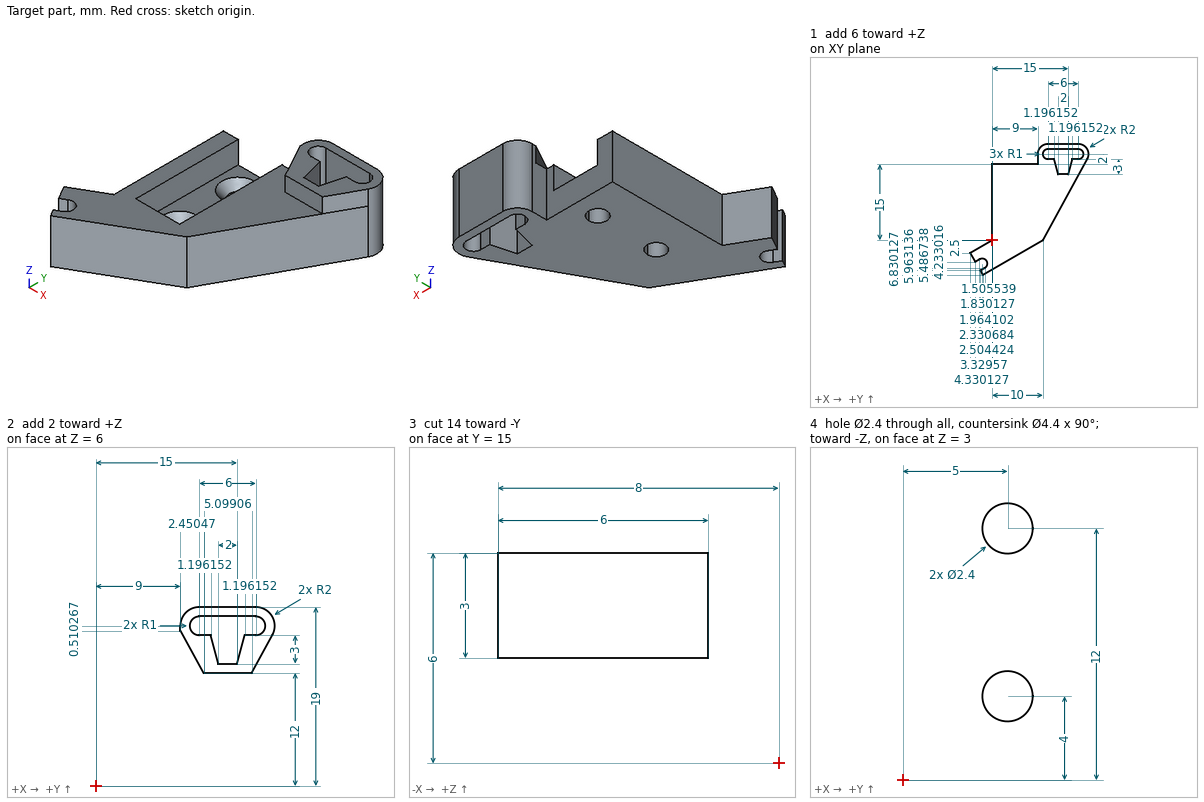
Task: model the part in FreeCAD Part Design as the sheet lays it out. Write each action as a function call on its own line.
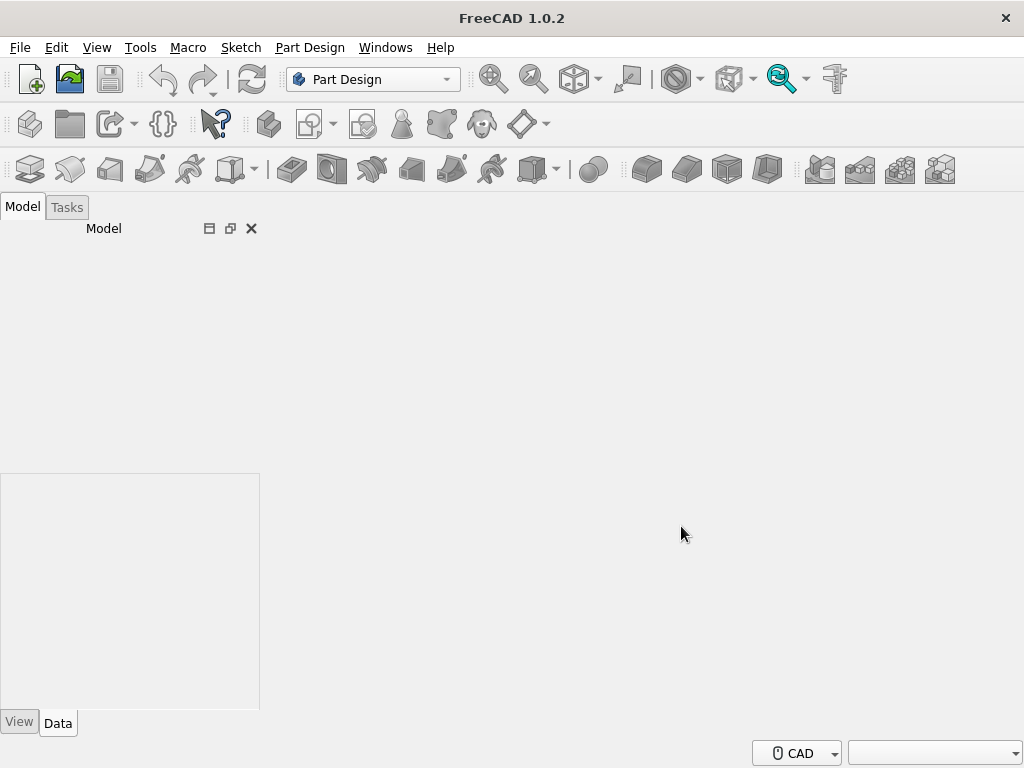
click(30, 80)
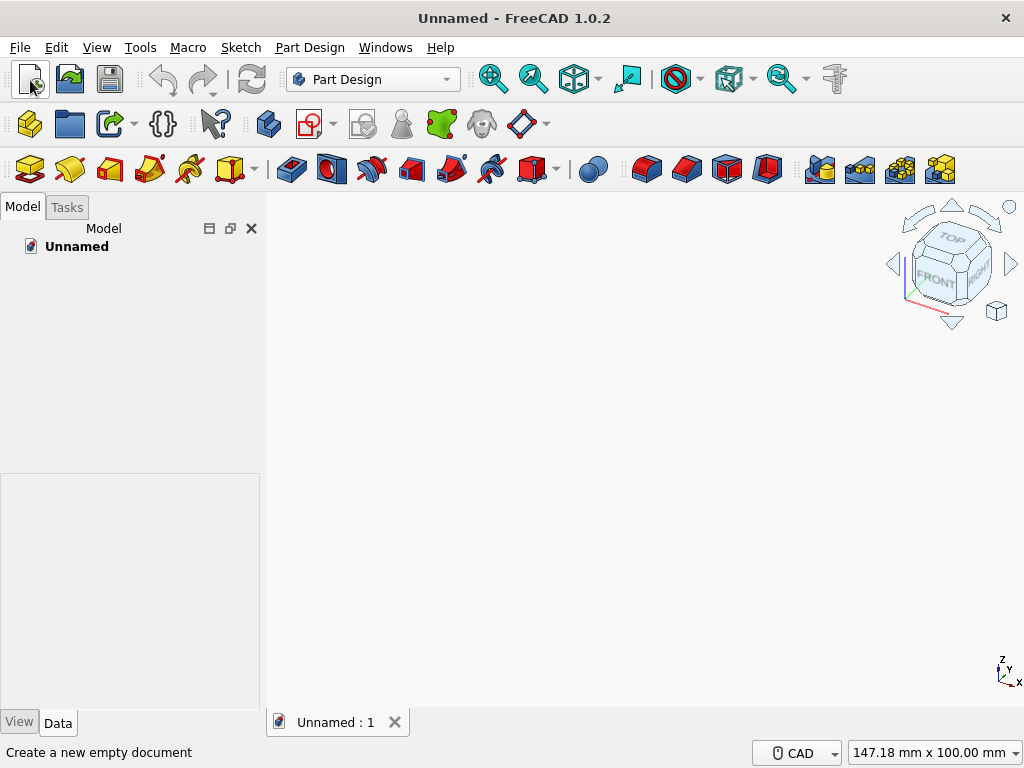
click(310, 124)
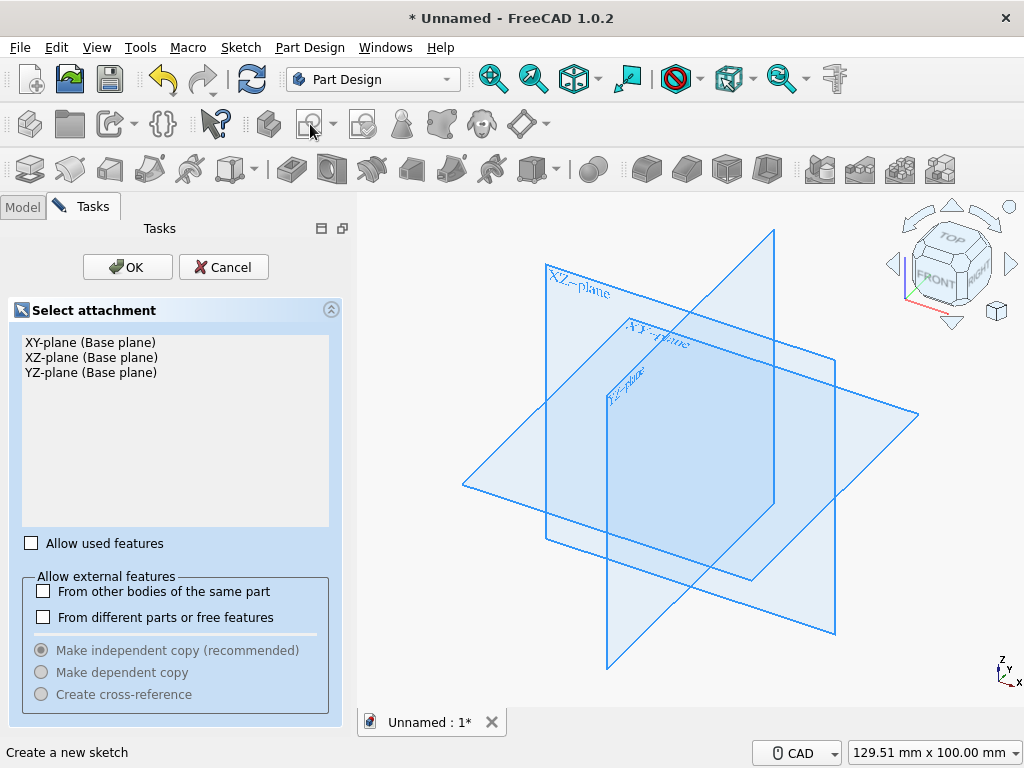
click(82, 342)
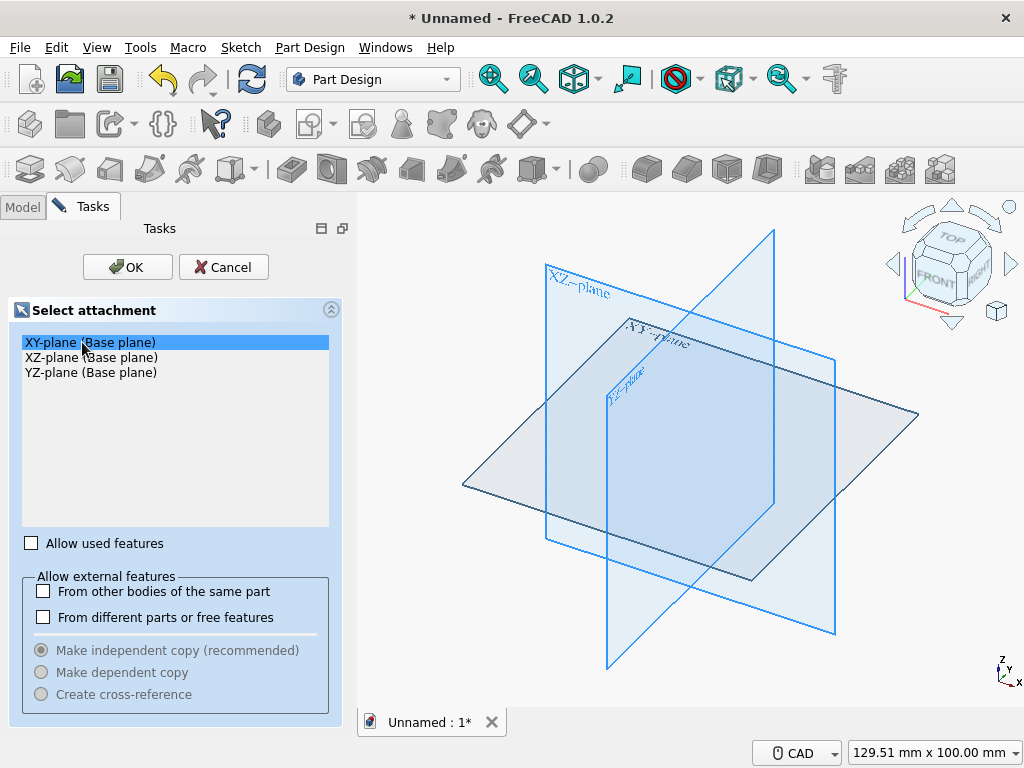
click(128, 267)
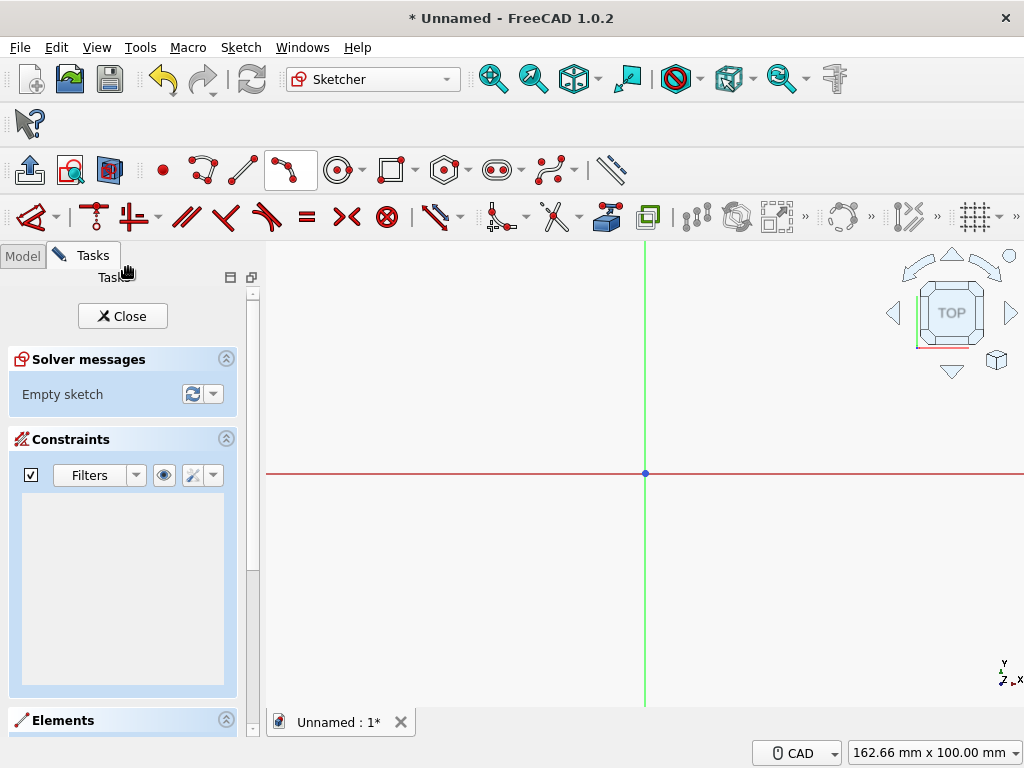
scroll(762, 423, up, 4)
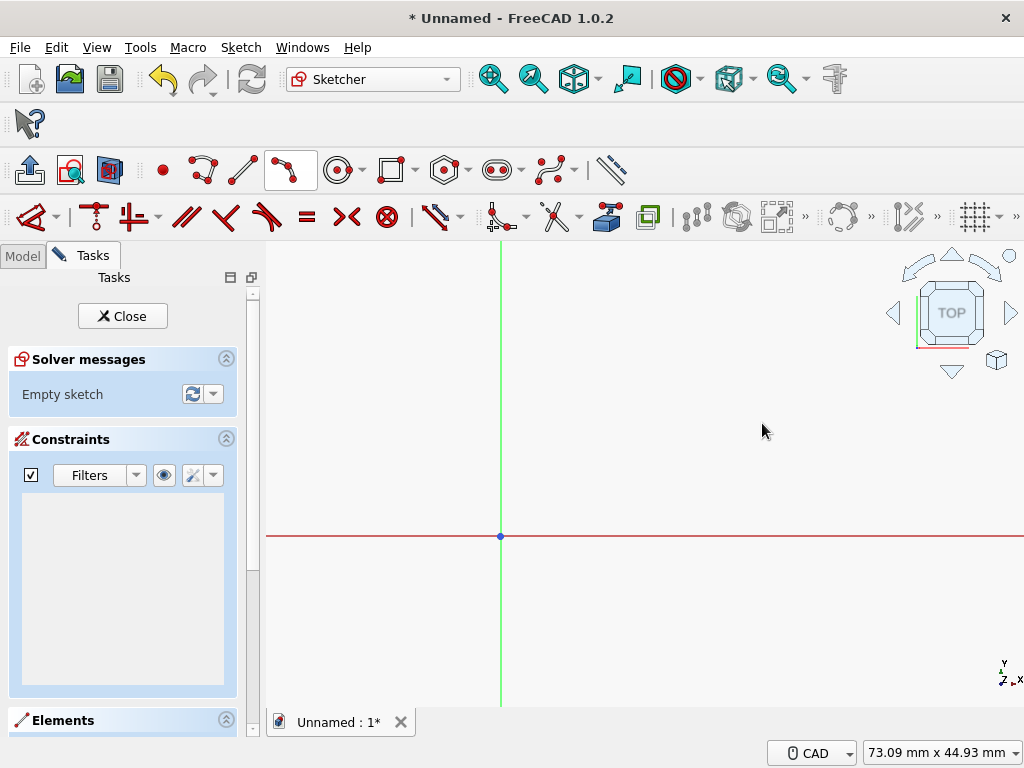
key(g)
key(m)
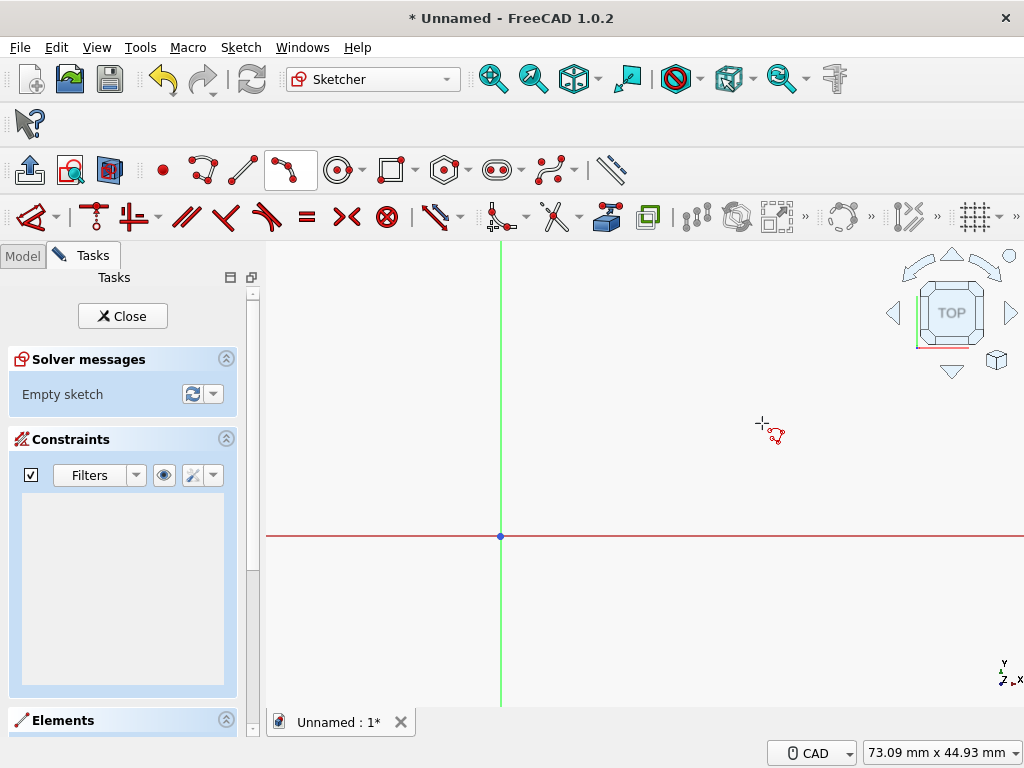
click(485, 593)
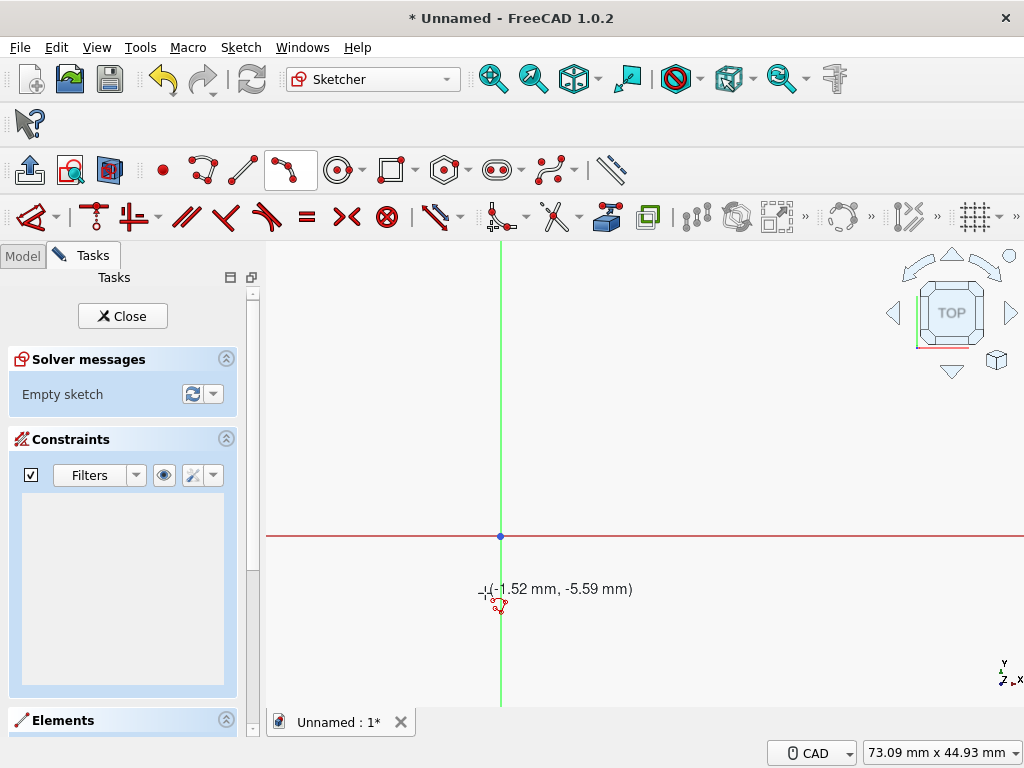
scroll(477, 598, up, 3)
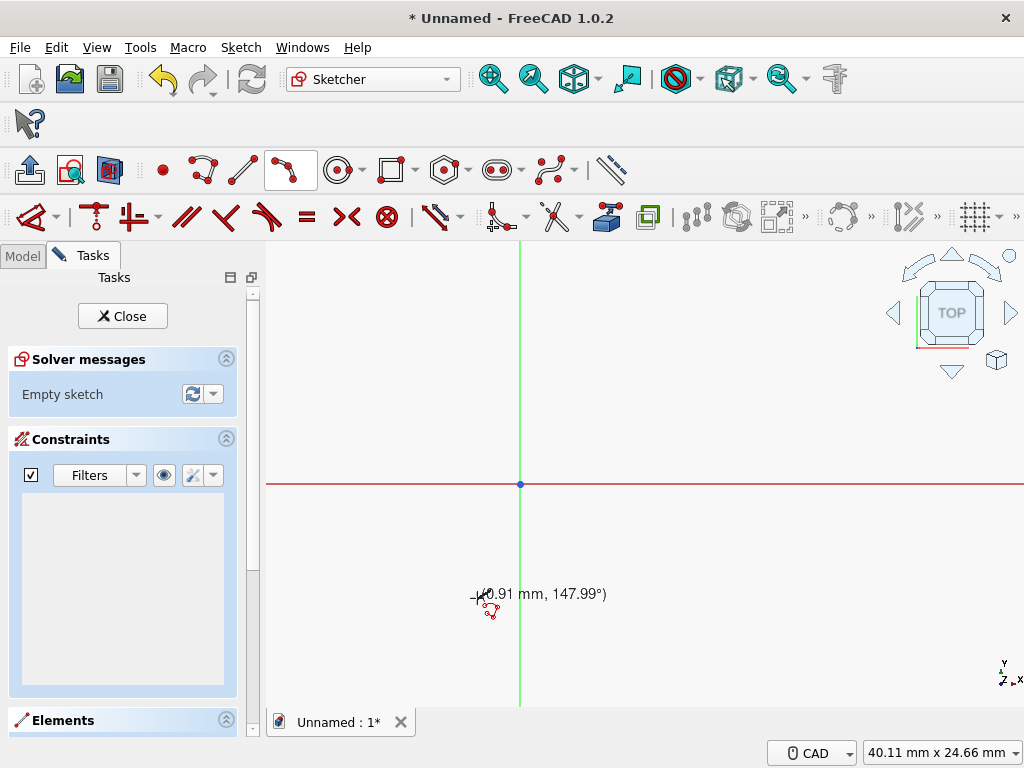
click(476, 597)
click(486, 614)
click(709, 484)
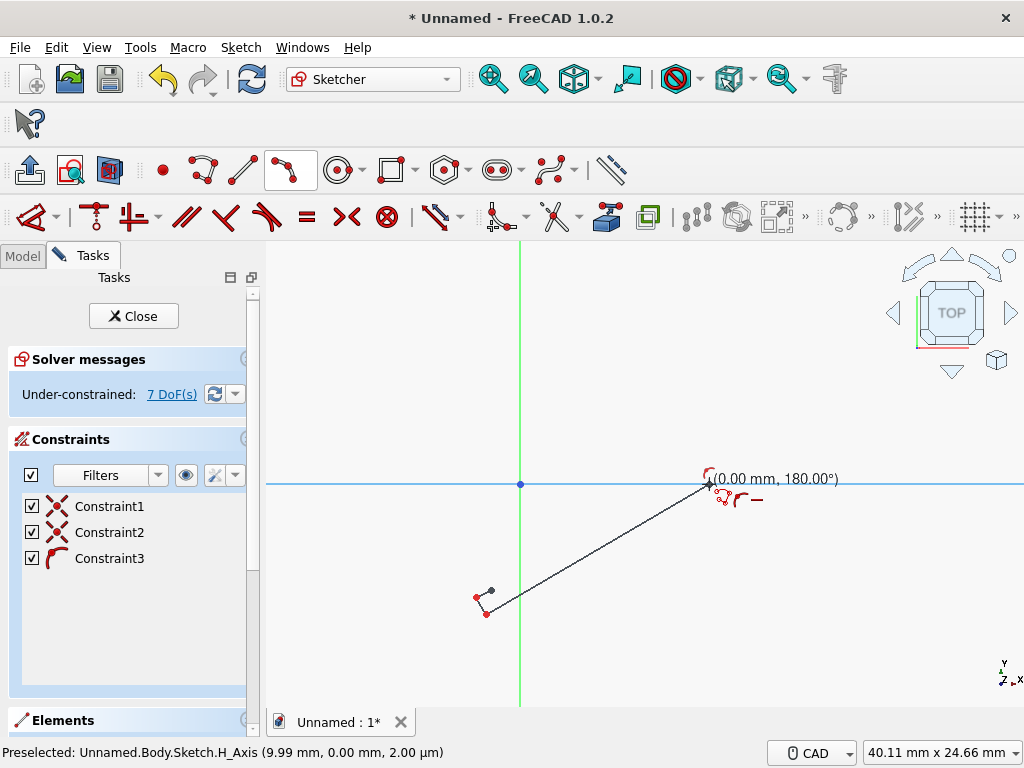
scroll(479, 601, down, 3)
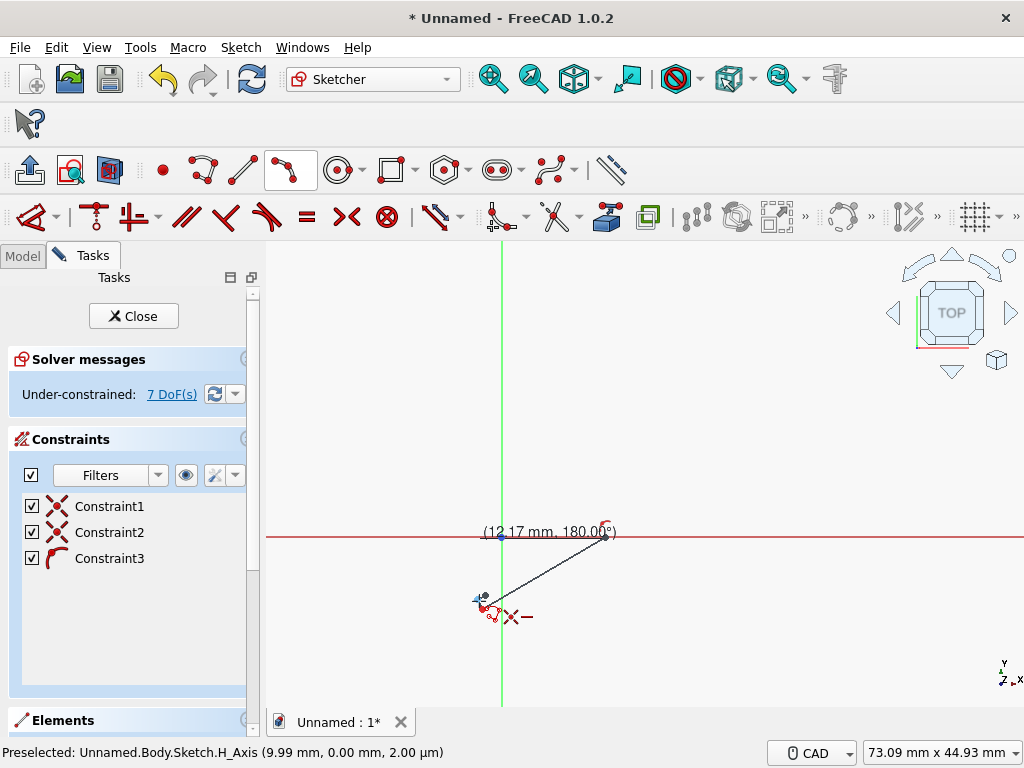
click(696, 371)
right_click(696, 371)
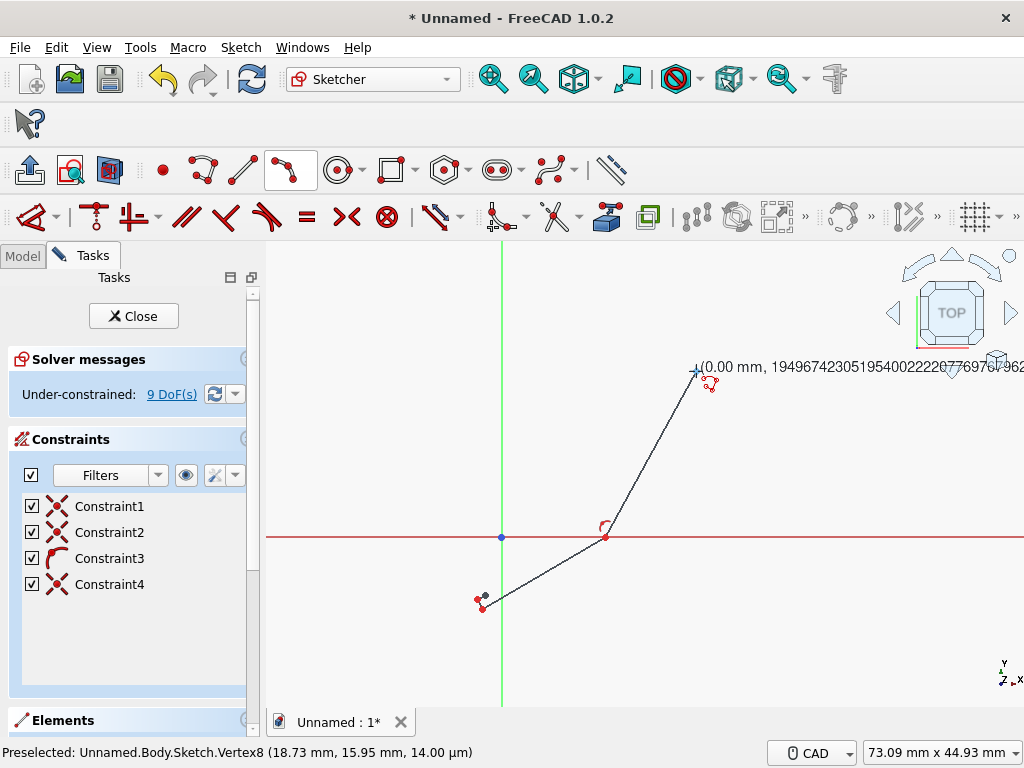
key(g)
key(l)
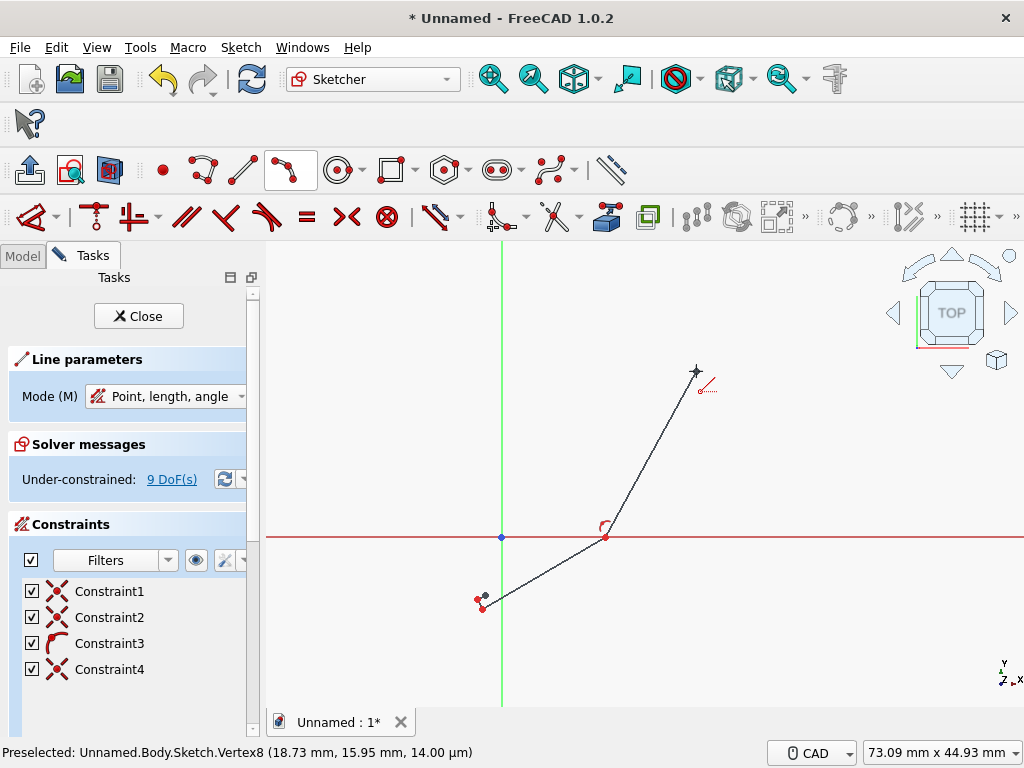
click(678, 340)
click(616, 340)